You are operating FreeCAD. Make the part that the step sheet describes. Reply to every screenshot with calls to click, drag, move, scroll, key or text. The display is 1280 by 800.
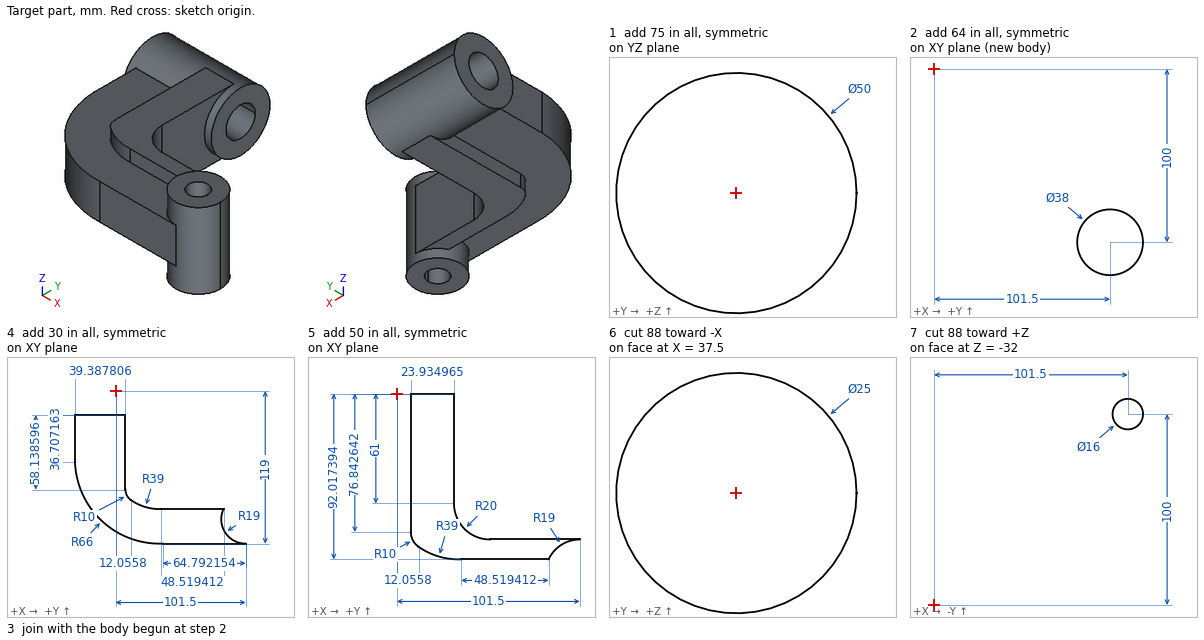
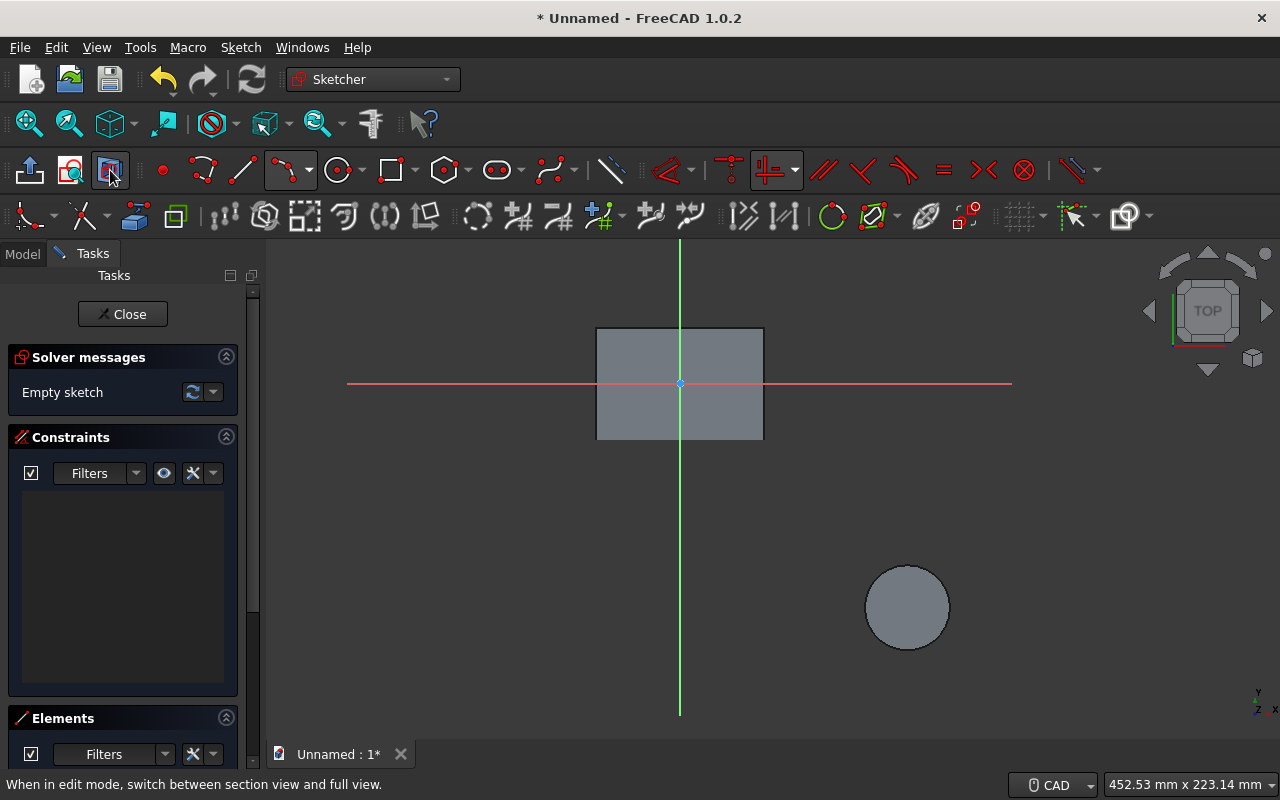
click(244, 170)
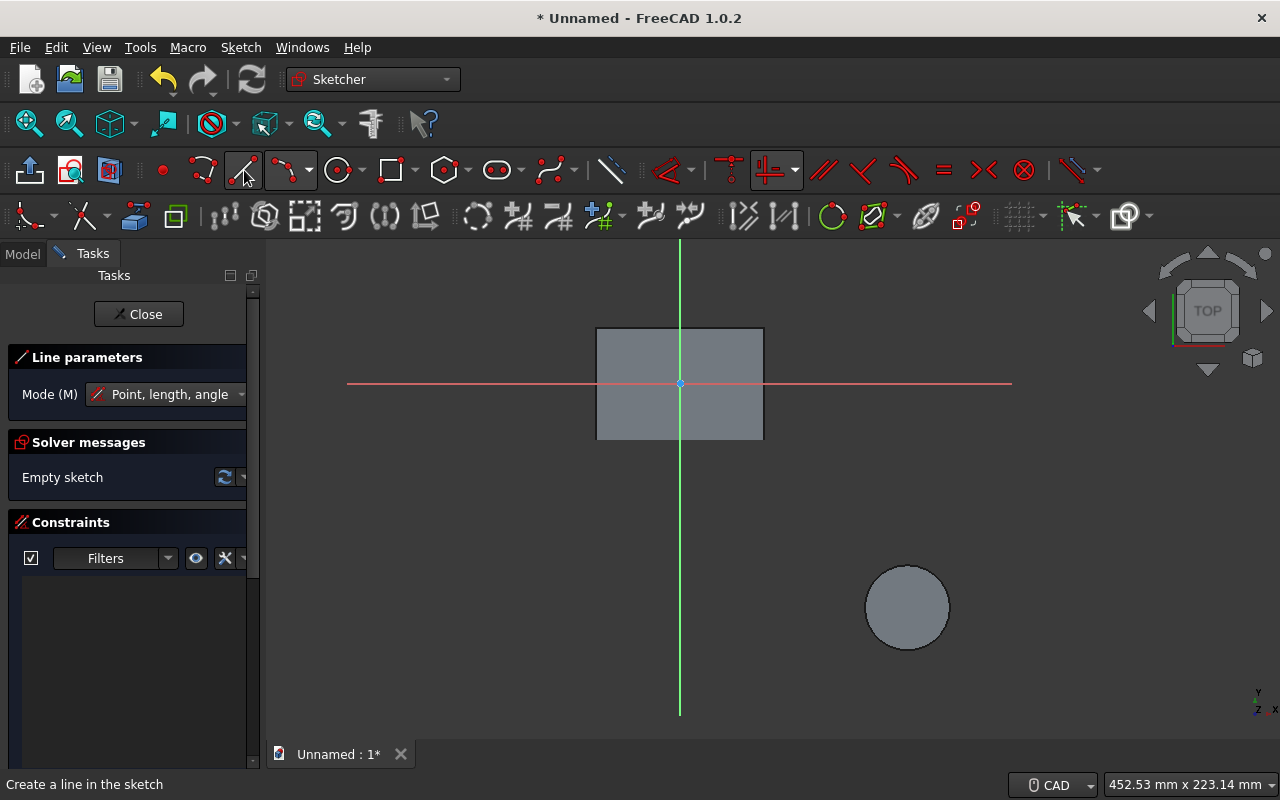
click(762, 650)
click(907, 650)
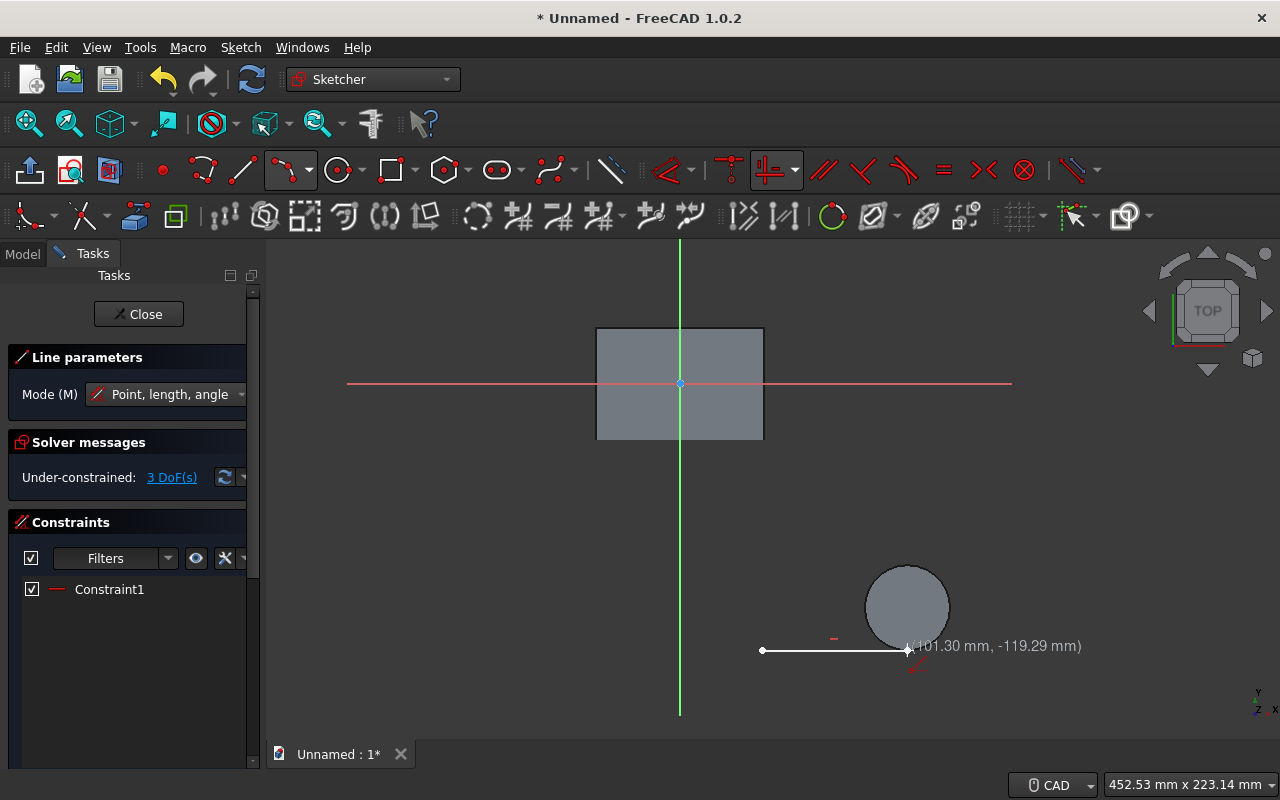
click(869, 590)
click(760, 590)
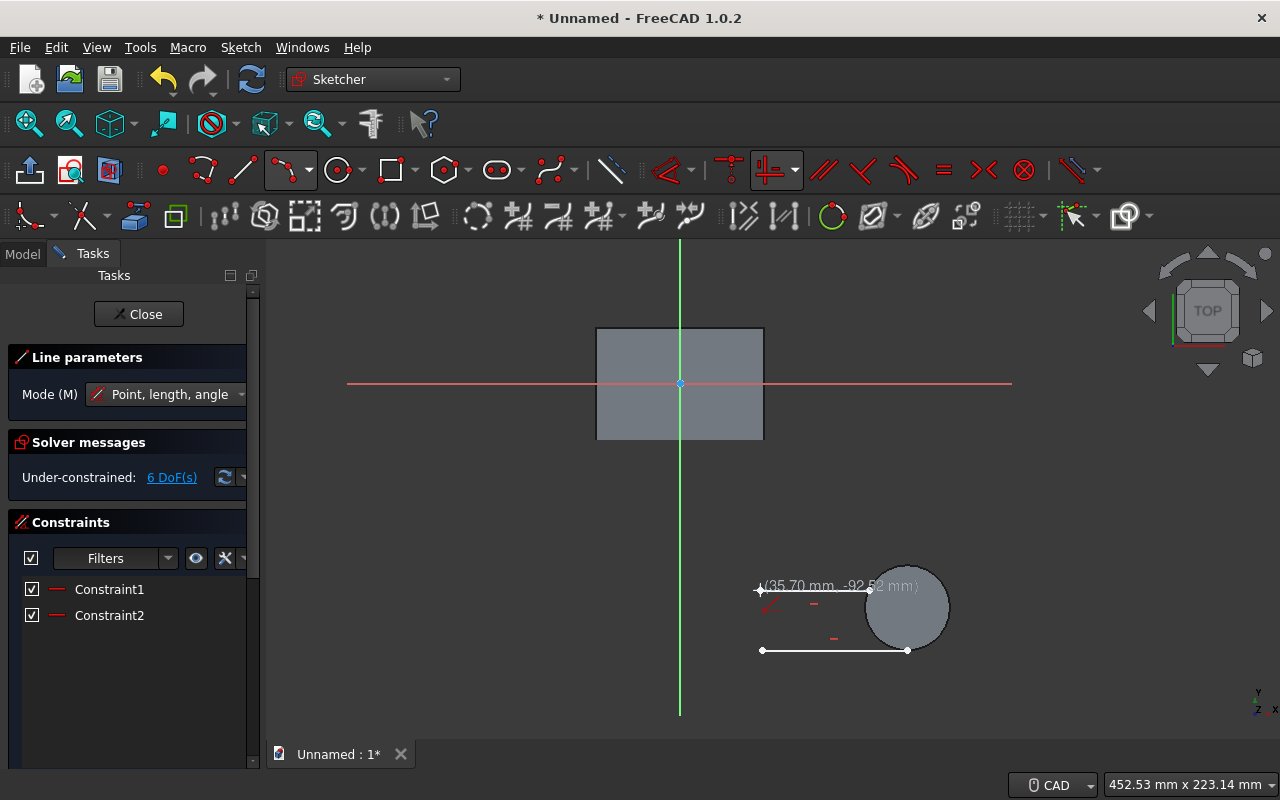
click(204, 170)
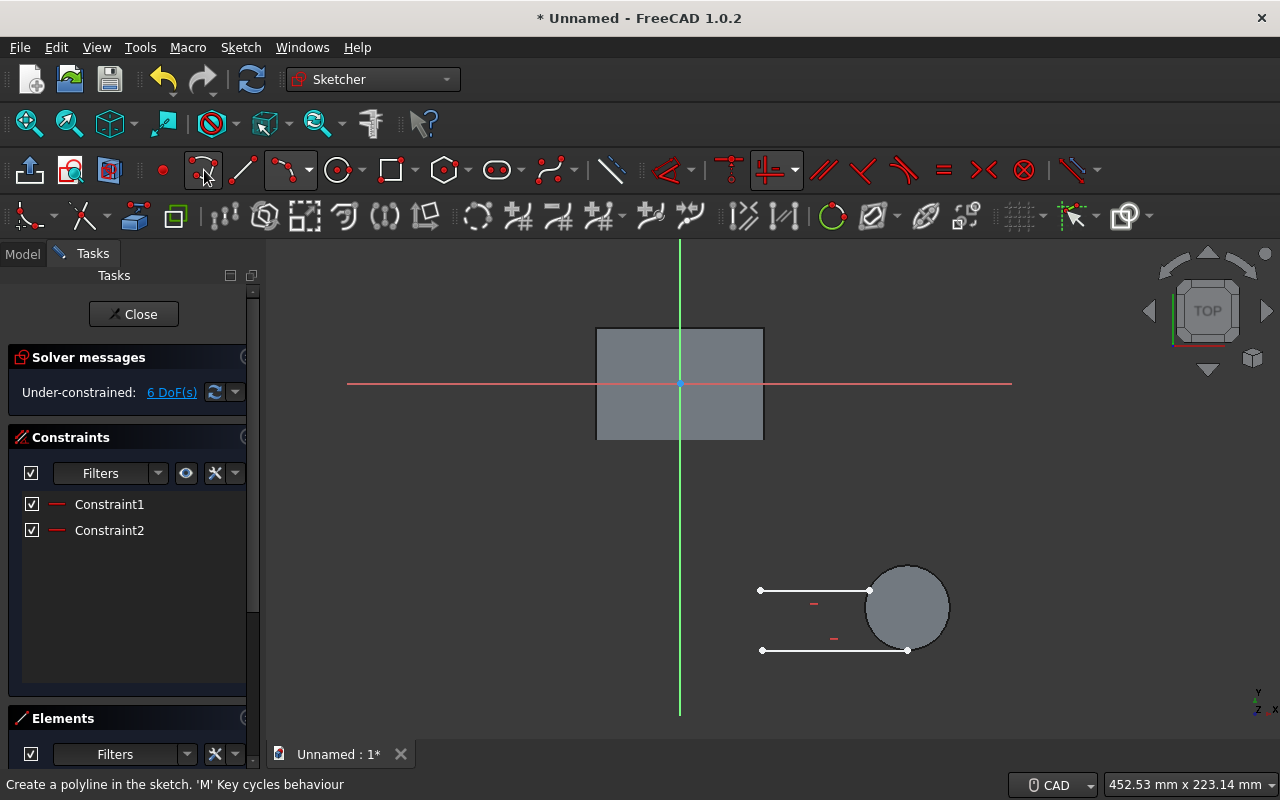
click(697, 556)
click(697, 426)
click(609, 426)
click(609, 508)
right_click(609, 508)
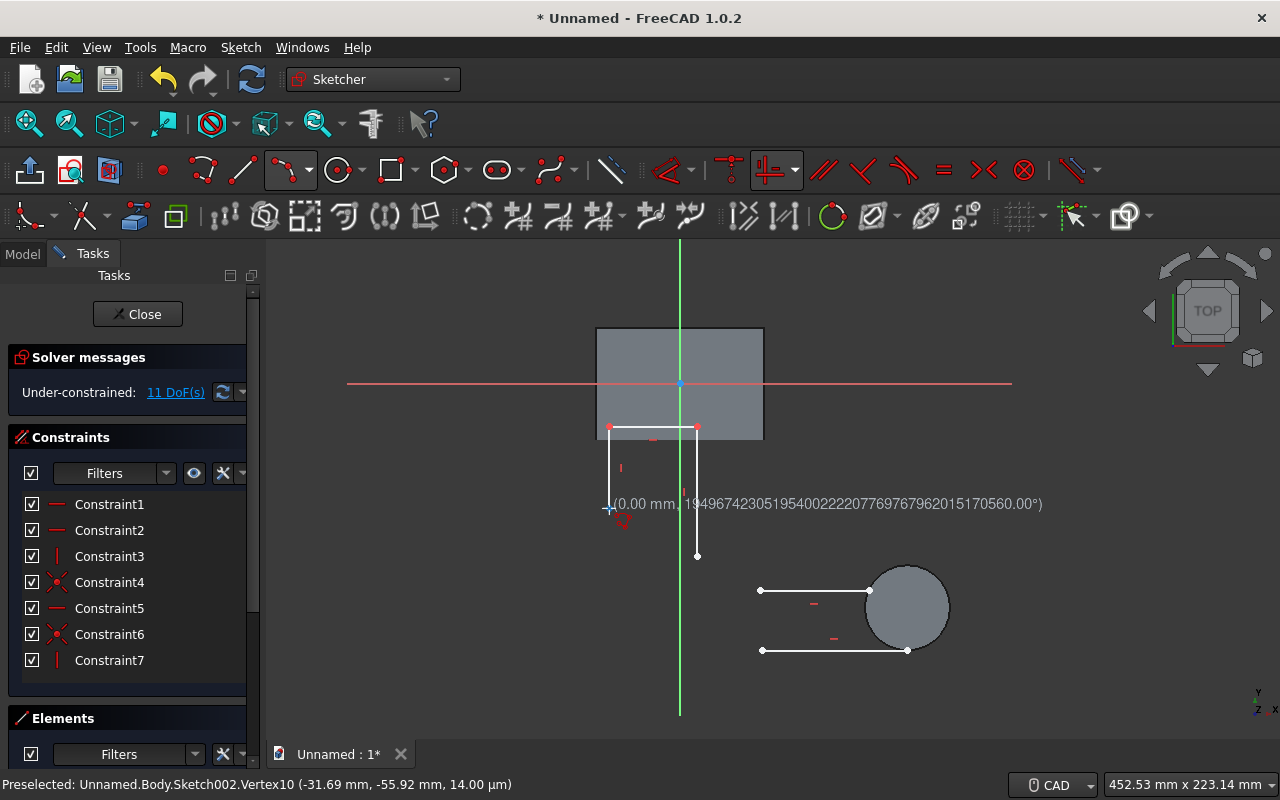
key(g)
key(3)
key(a)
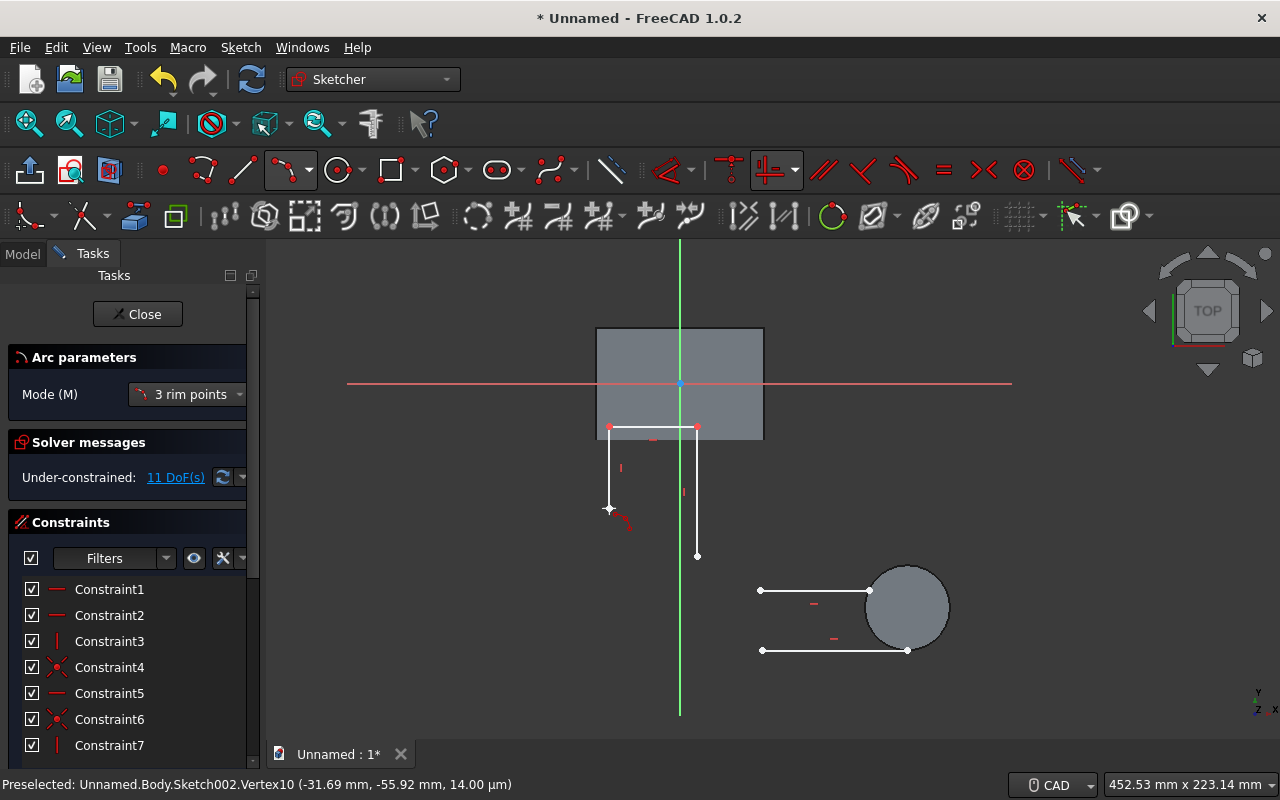
click(907, 651)
click(869, 591)
click(872, 631)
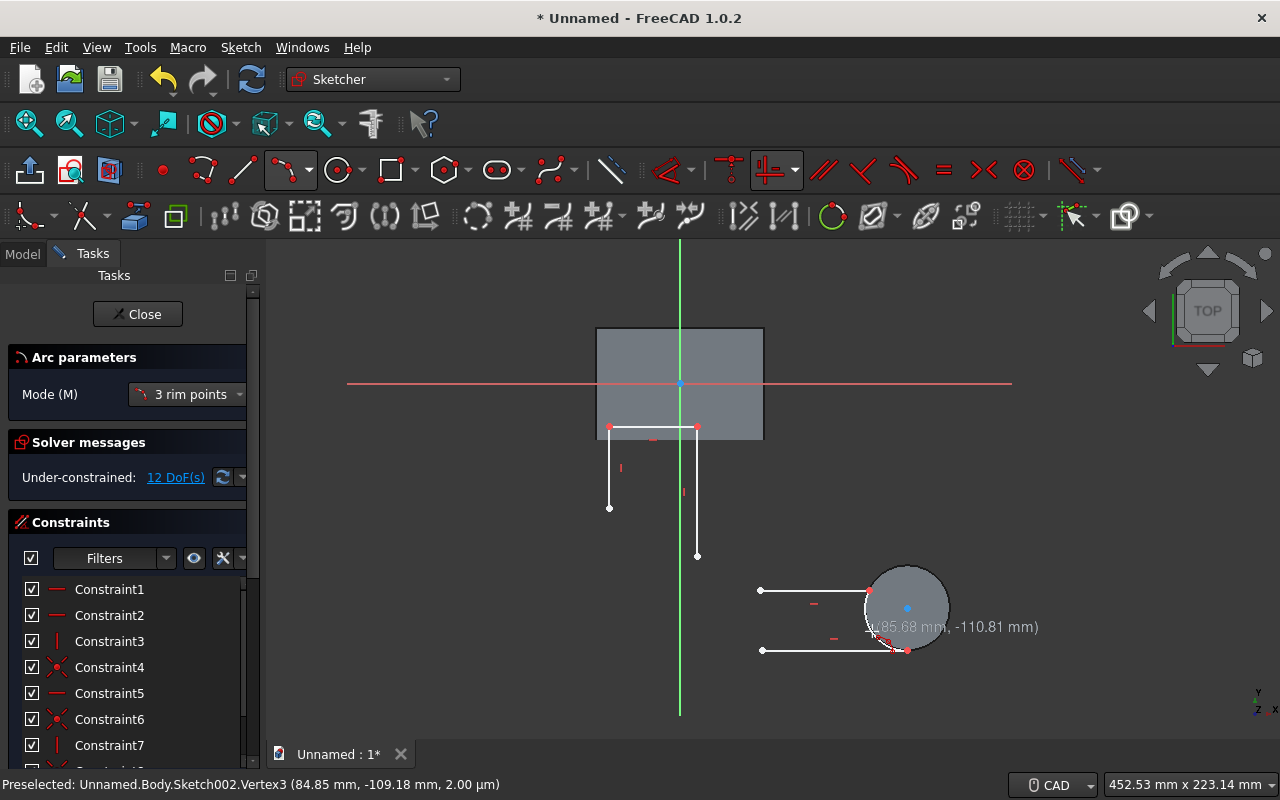
click(760, 591)
click(707, 574)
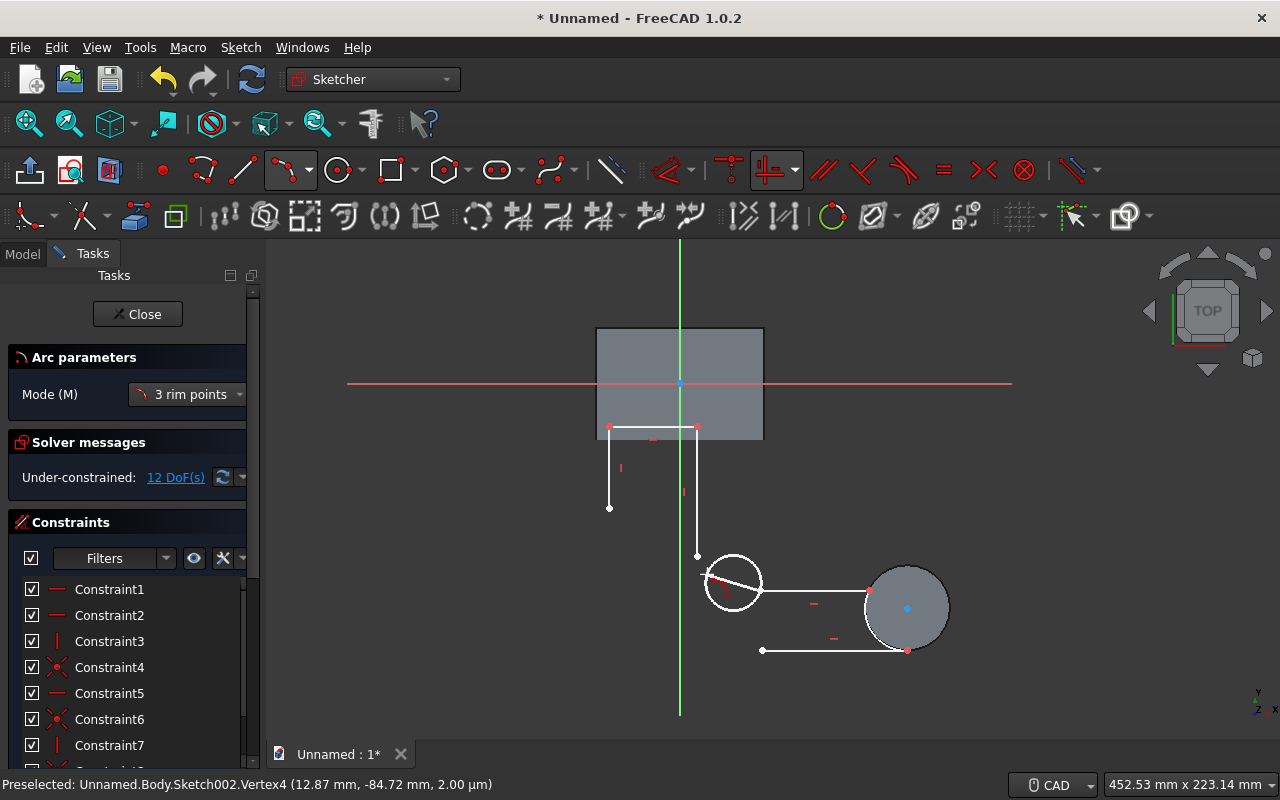
scroll(732, 586, up, 7)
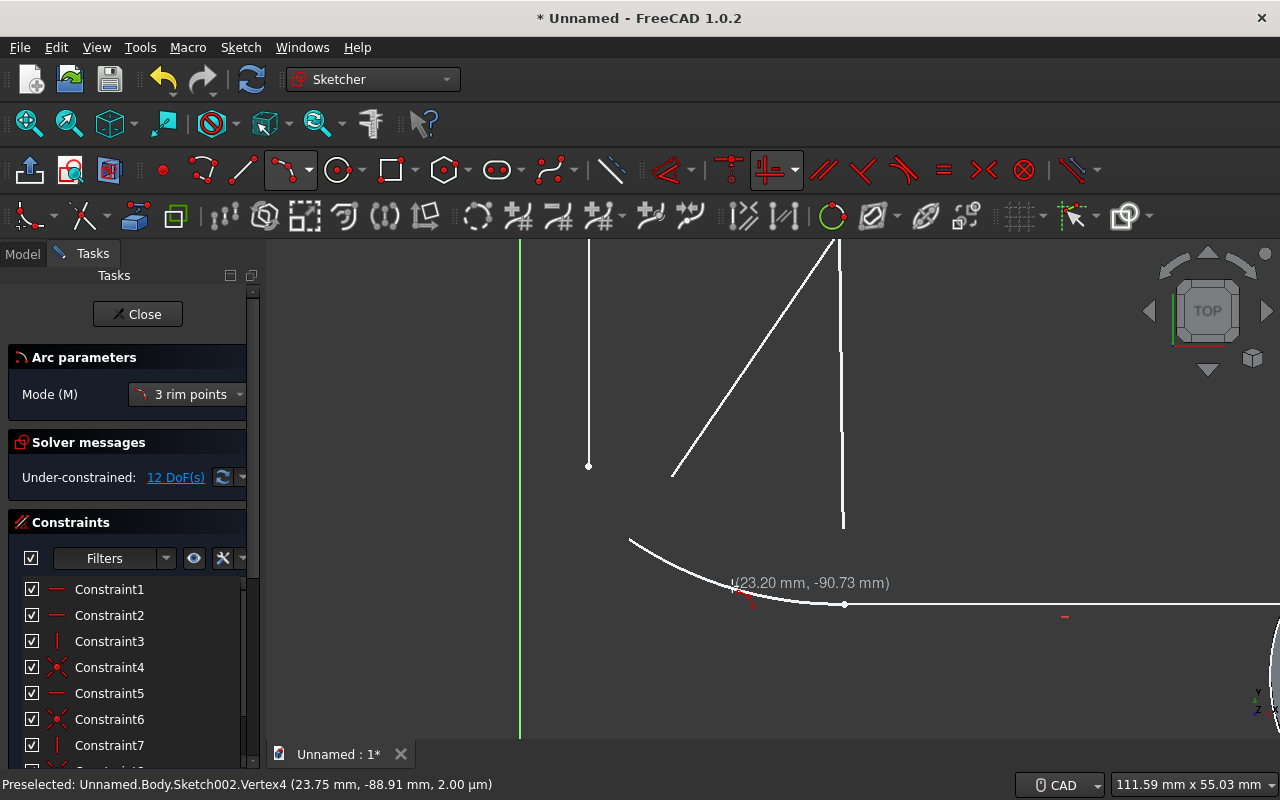
click(732, 585)